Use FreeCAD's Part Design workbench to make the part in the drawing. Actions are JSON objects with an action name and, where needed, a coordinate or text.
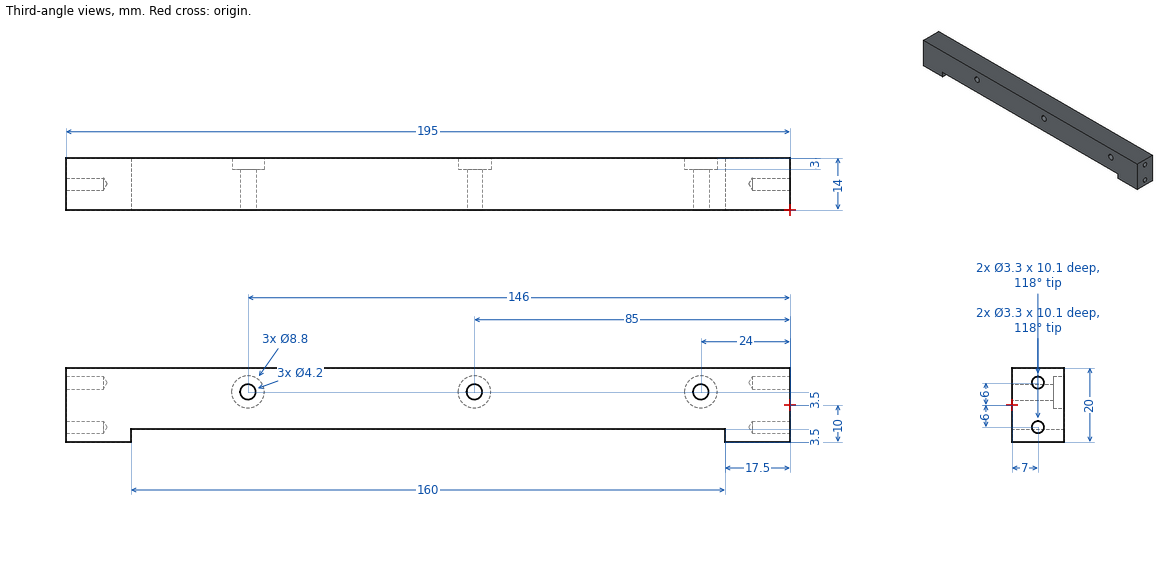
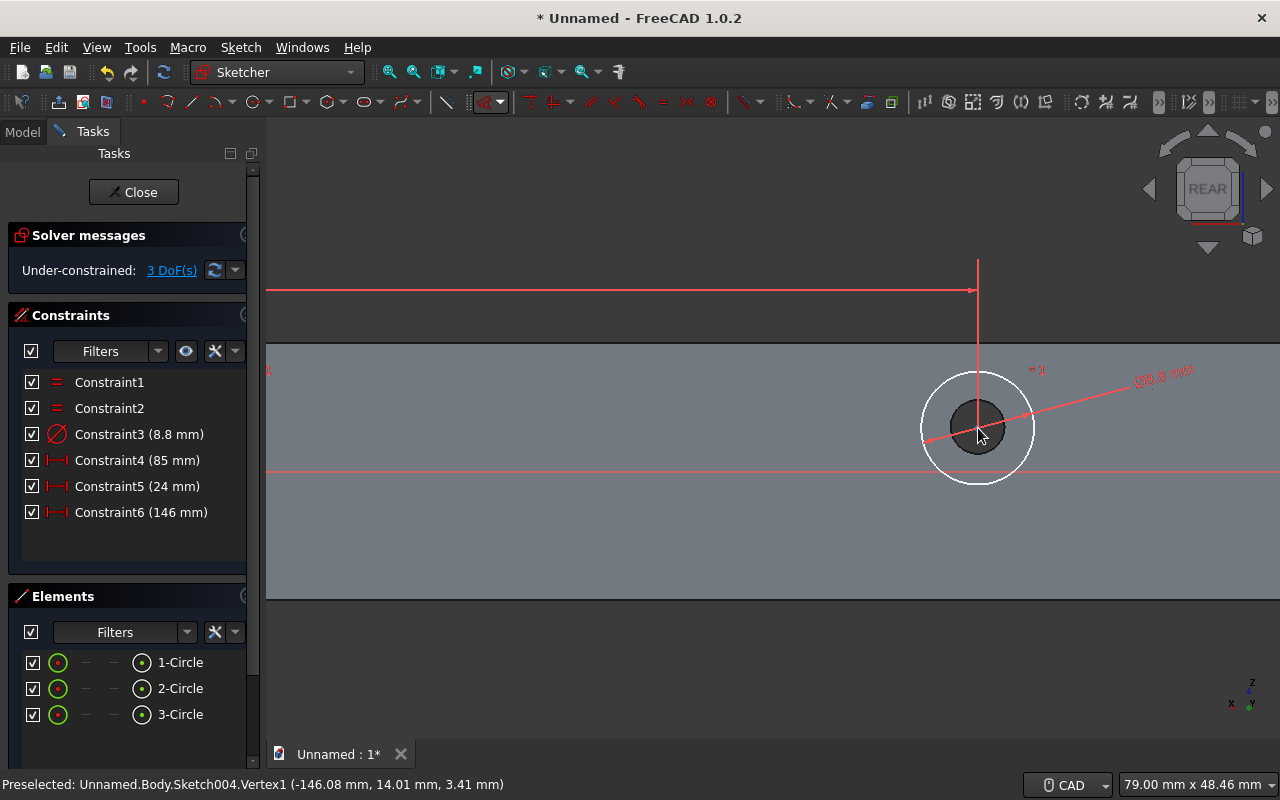
{"action": "left_click", "coordinate": [978, 428]}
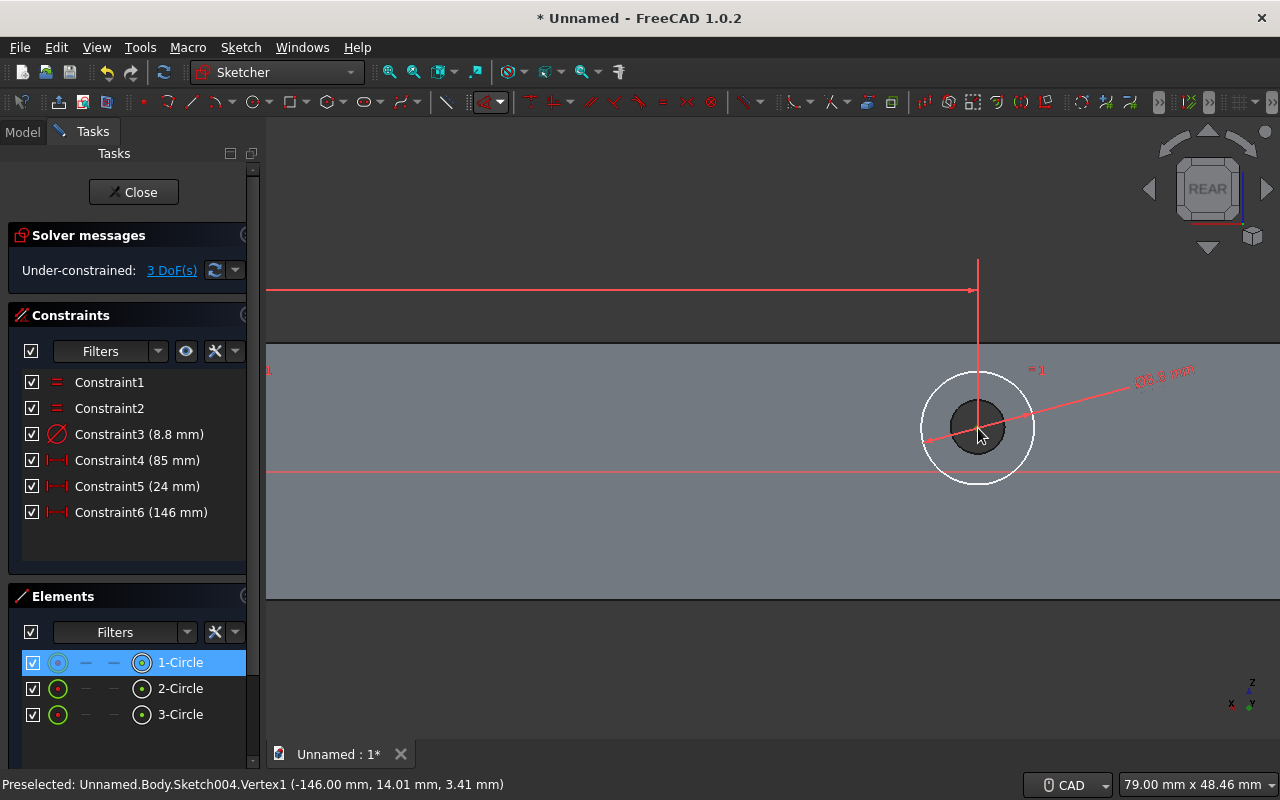
{"action": "key", "text": "i"}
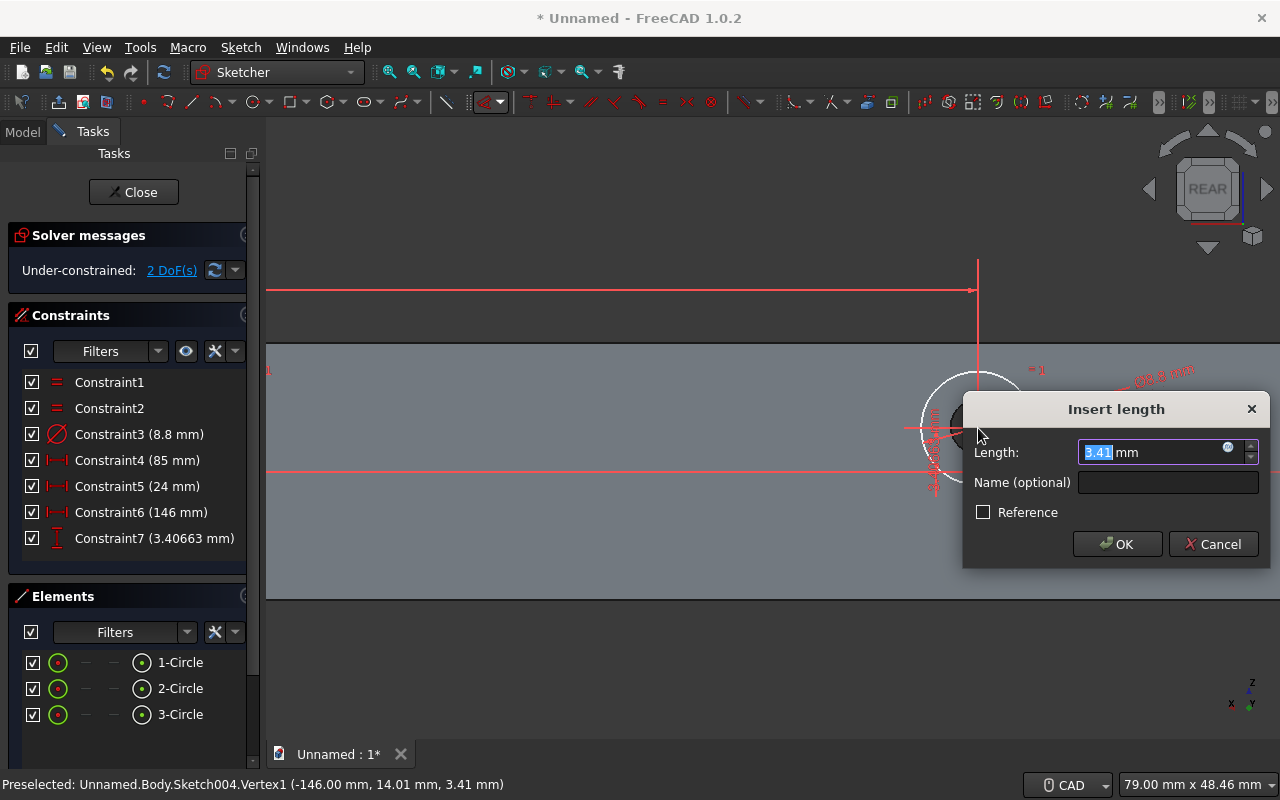
{"action": "type", "text": "3.5"}
{"action": "key", "text": "Return"}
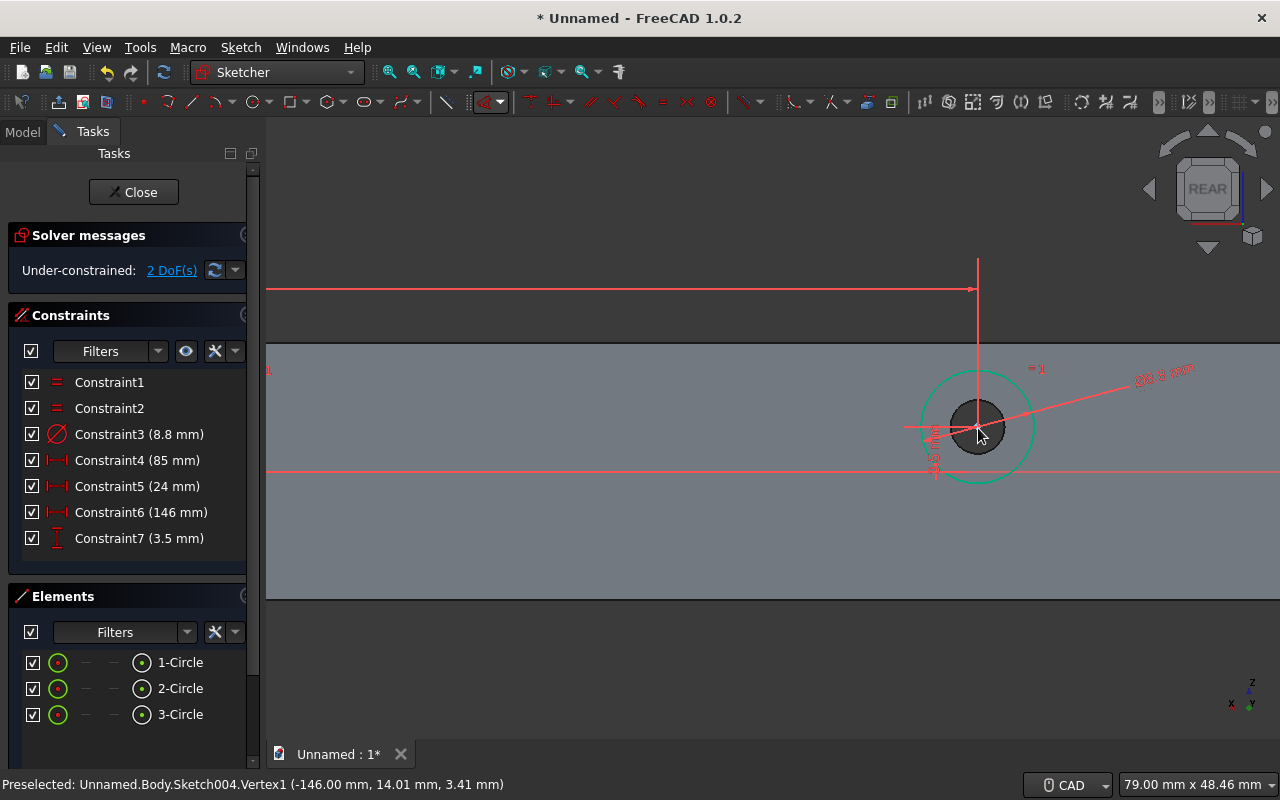
{"action": "scroll", "coordinate": [978, 428], "scroll_direction": "down", "scroll_amount": 6}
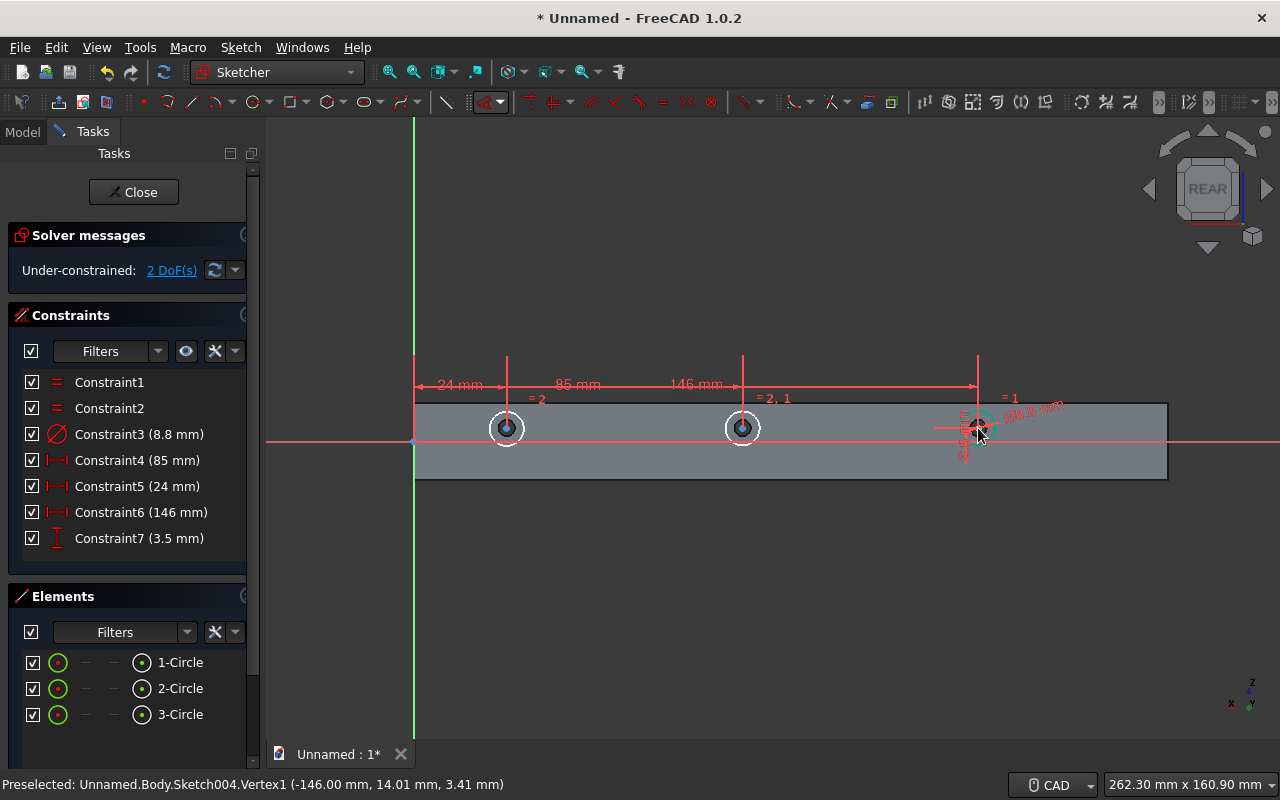
{"action": "scroll", "coordinate": [743, 428], "scroll_direction": "up", "scroll_amount": 6}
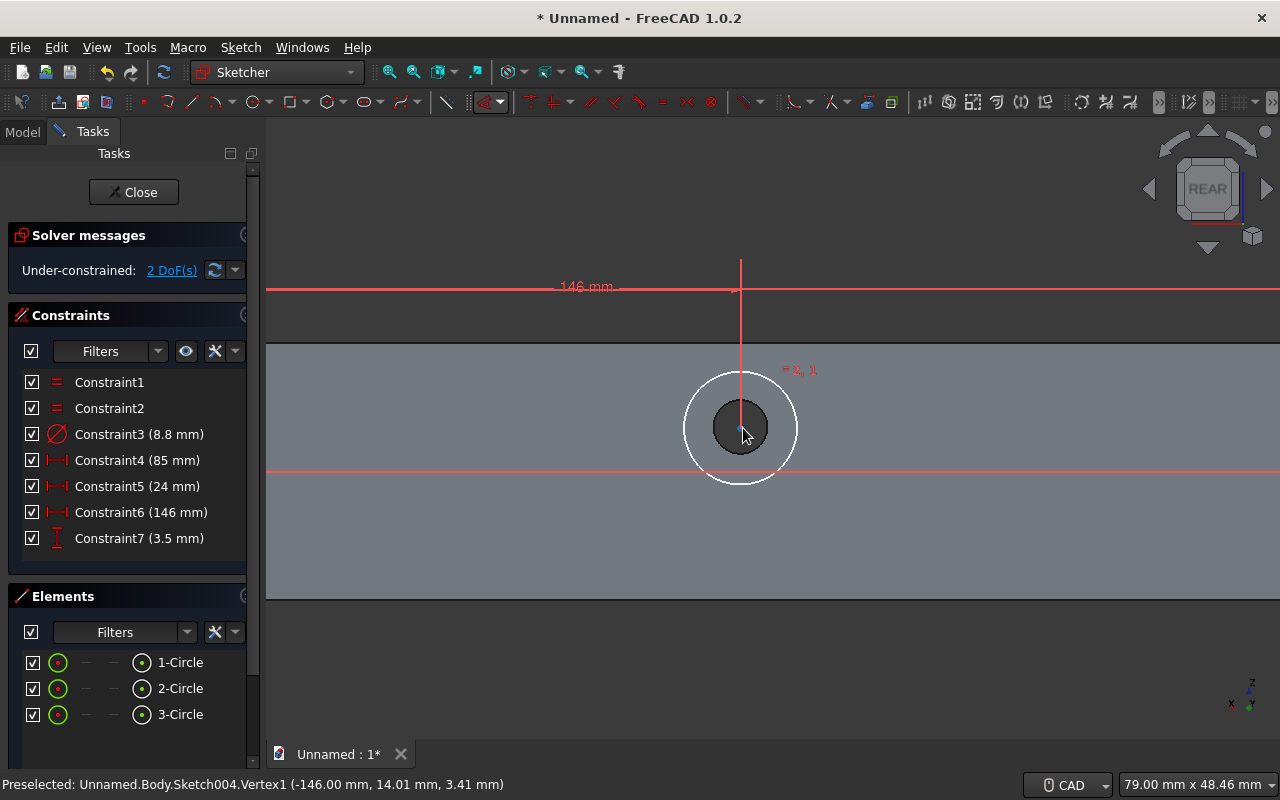
{"action": "left_click", "coordinate": [741, 428]}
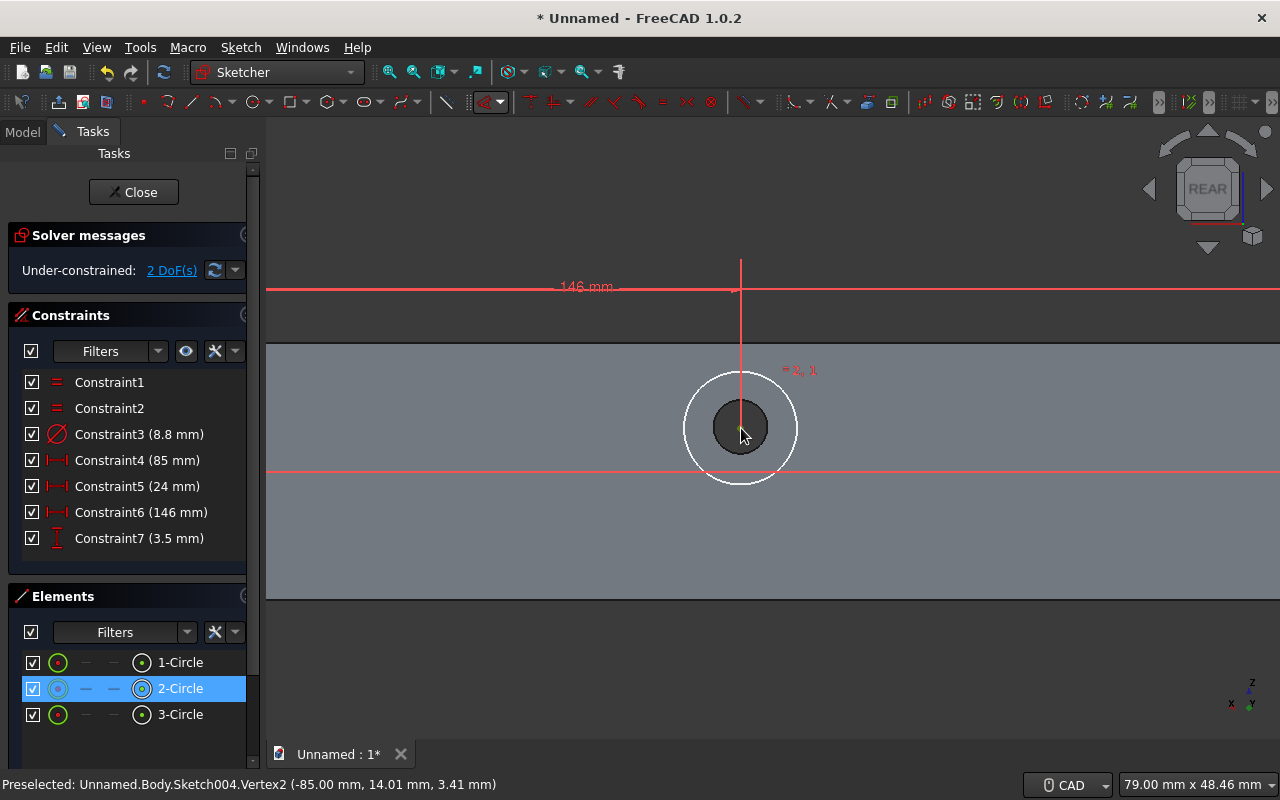
{"action": "key", "text": "i"}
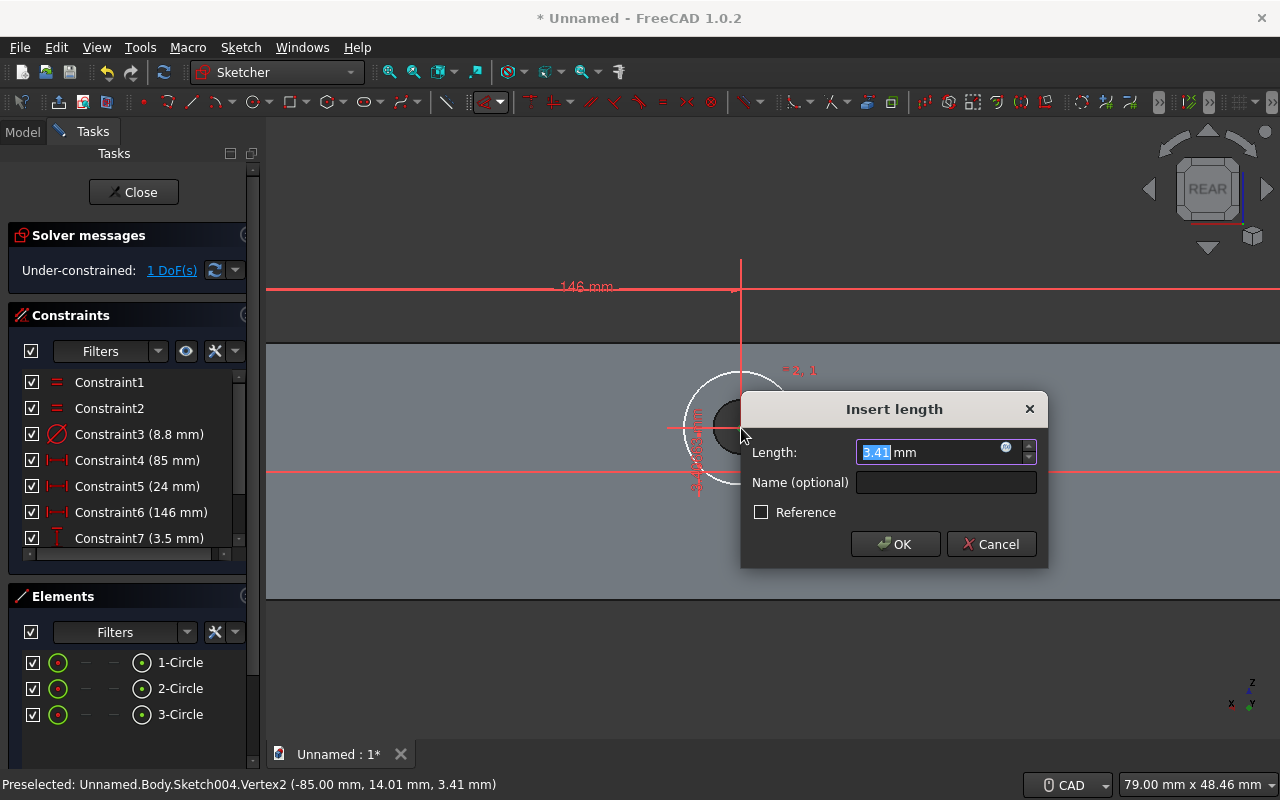
{"action": "type", "text": "3.5"}
{"action": "key", "text": "Return"}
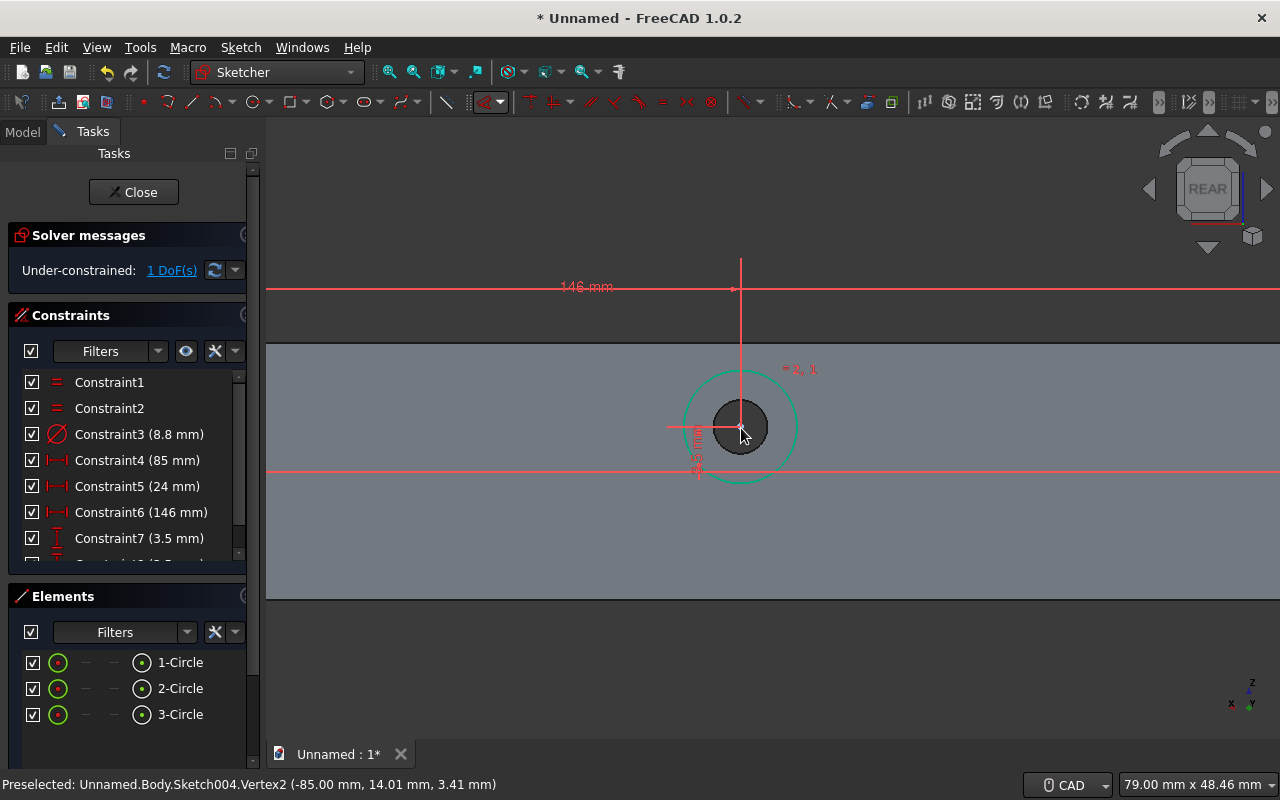
{"action": "scroll", "coordinate": [743, 428], "scroll_direction": "down", "scroll_amount": 6}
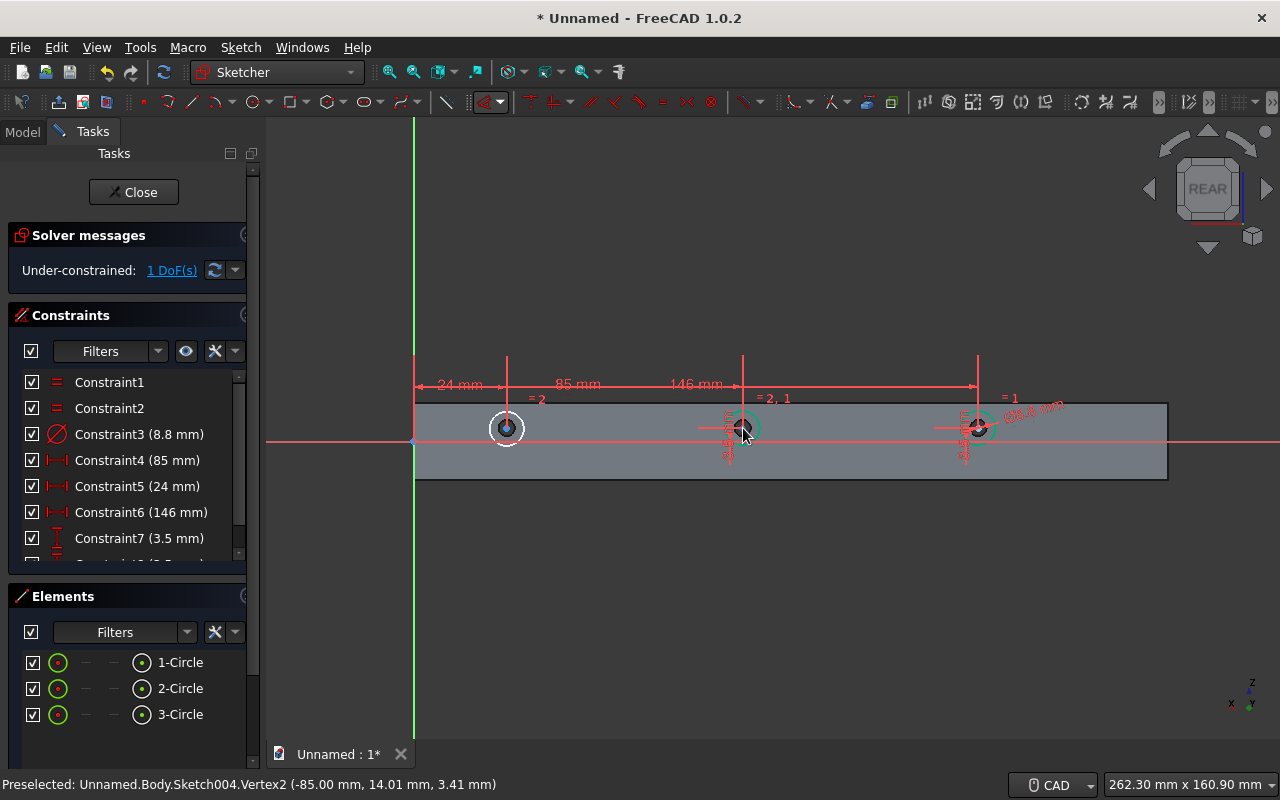
{"action": "scroll", "coordinate": [507, 429], "scroll_direction": "up", "scroll_amount": 6}